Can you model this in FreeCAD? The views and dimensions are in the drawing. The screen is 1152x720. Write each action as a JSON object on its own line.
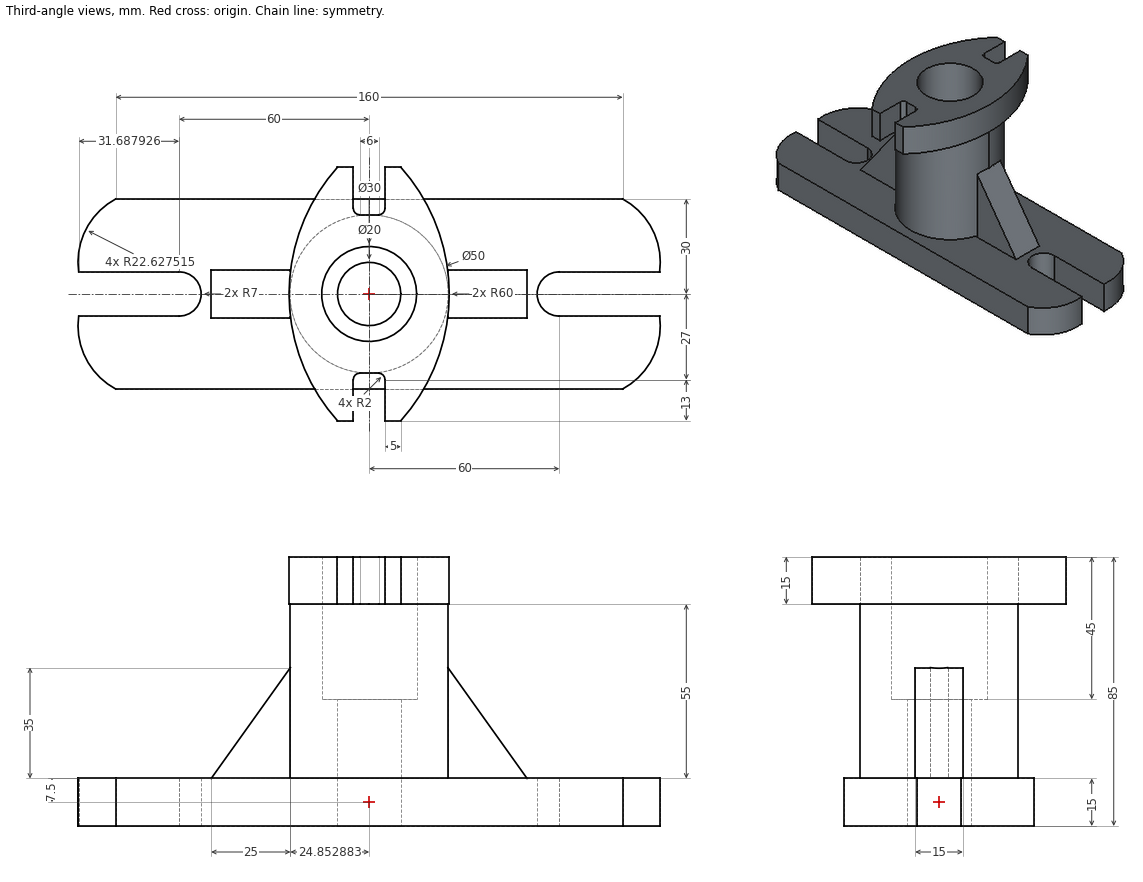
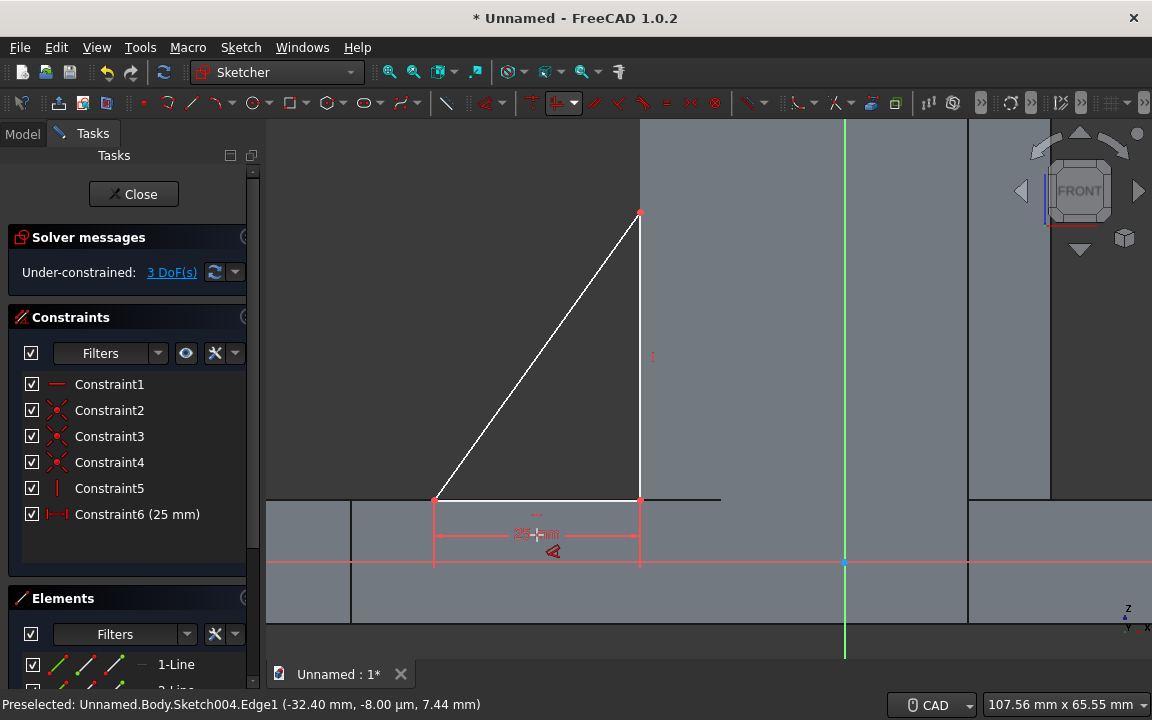
{"action": "left_click", "coordinate": [640, 299]}
{"action": "left_click", "coordinate": [674, 357]}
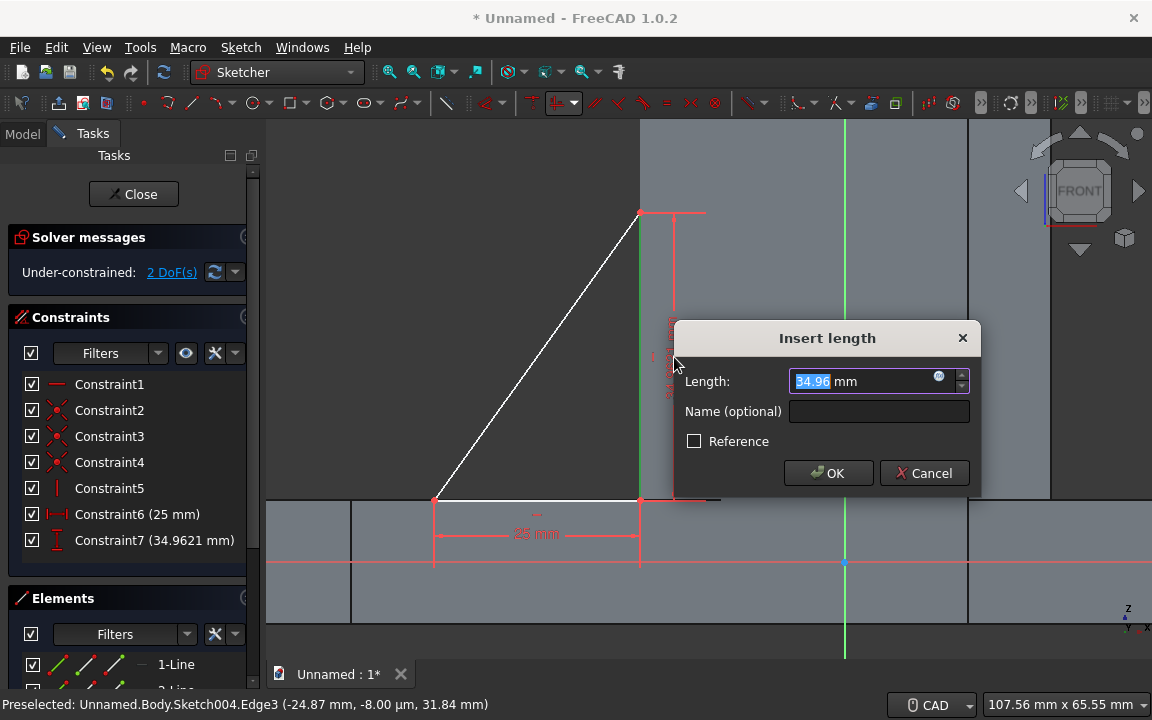
{"action": "type", "text": "35"}
{"action": "key", "text": "Return"}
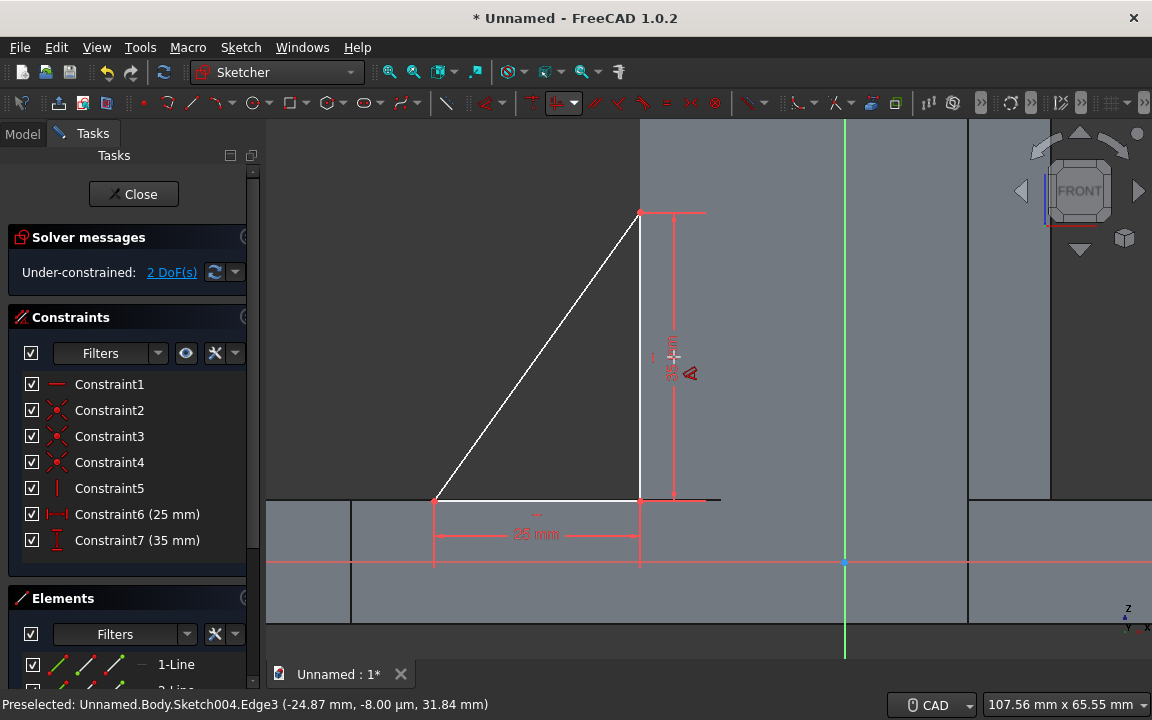
{"action": "left_click", "coordinate": [640, 501]}
{"action": "left_click", "coordinate": [879, 532]}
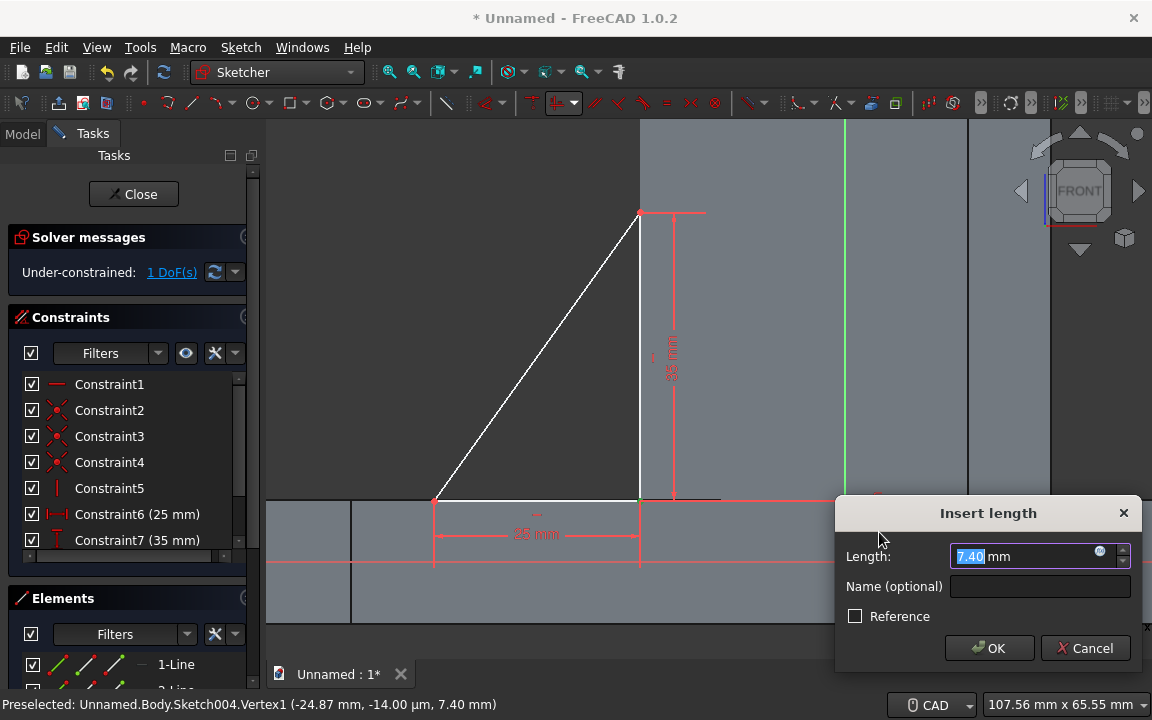
{"action": "type", "text": "7.5"}
{"action": "key", "text": "Return"}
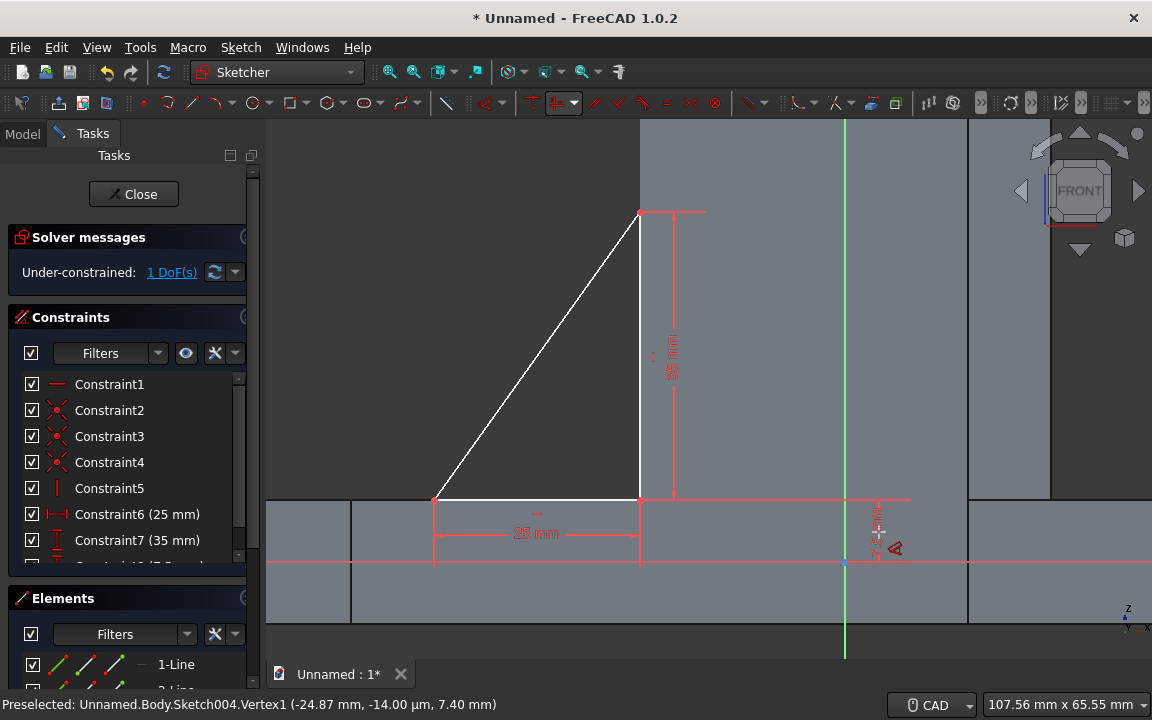
{"action": "left_click", "coordinate": [640, 500]}
{"action": "left_click", "coordinate": [742, 596]}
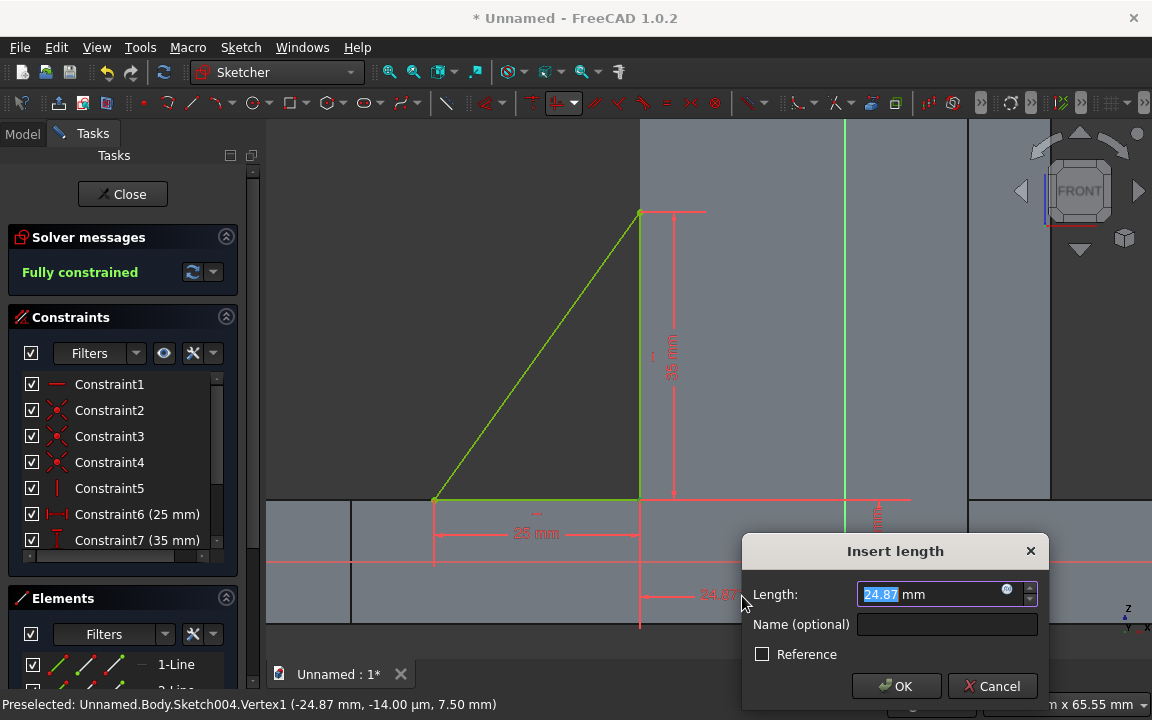
{"action": "type", "text": "24.852883"}
{"action": "key", "text": "Return"}
{"action": "key", "text": "Escape"}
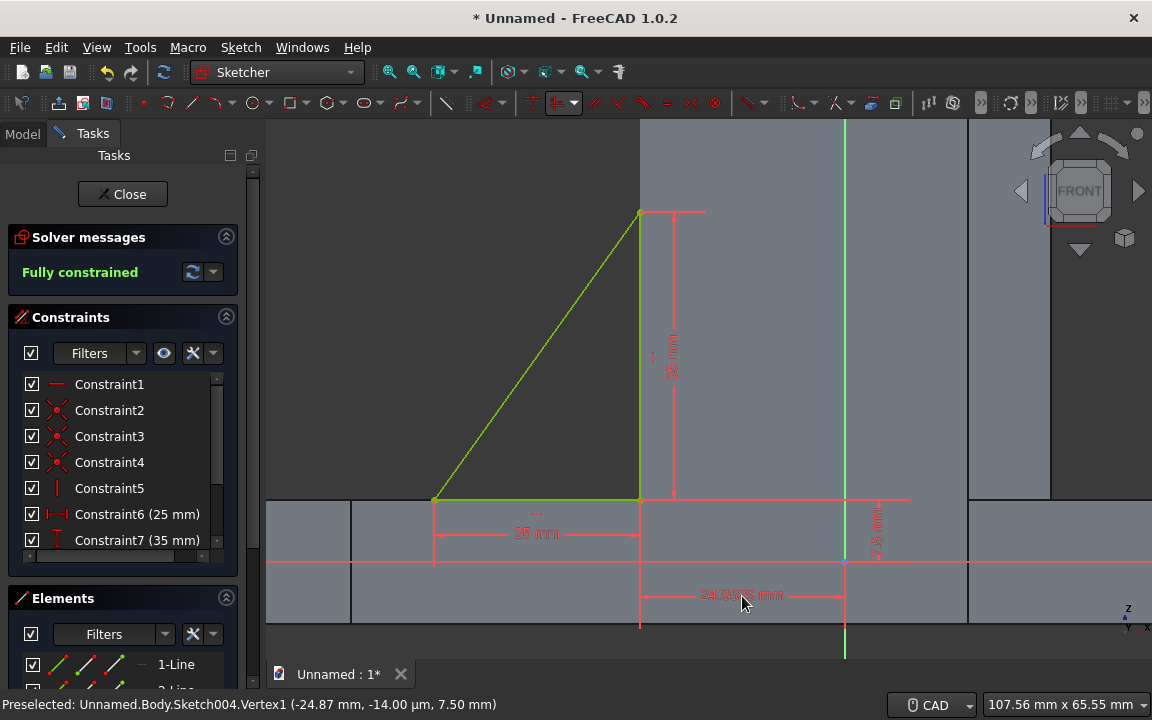
{"action": "left_click", "coordinate": [123, 194]}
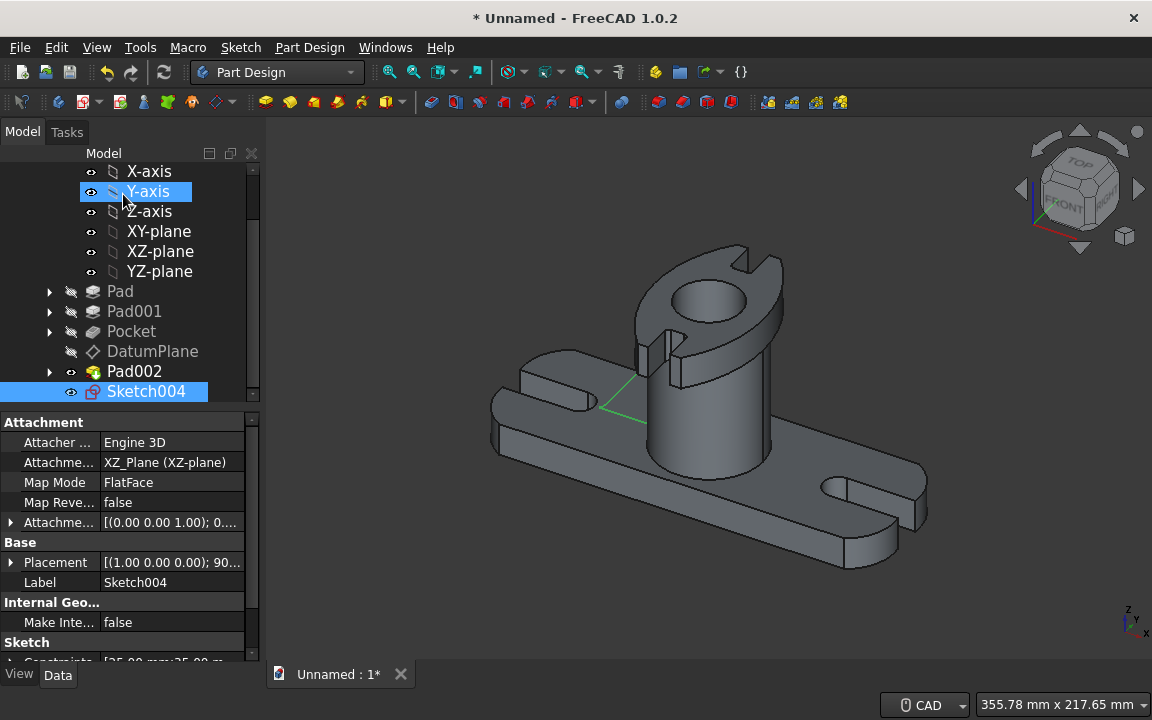
{"action": "left_click", "coordinate": [266, 102]}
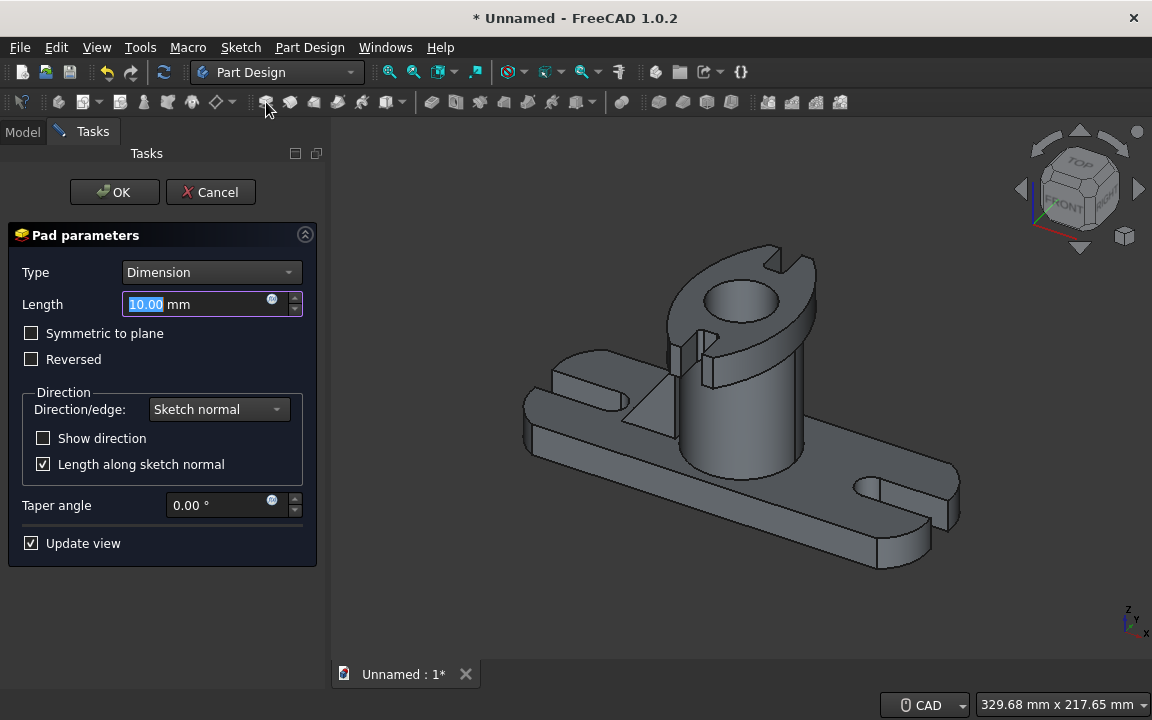
{"action": "type", "text": "15"}
{"action": "key", "text": "Tab"}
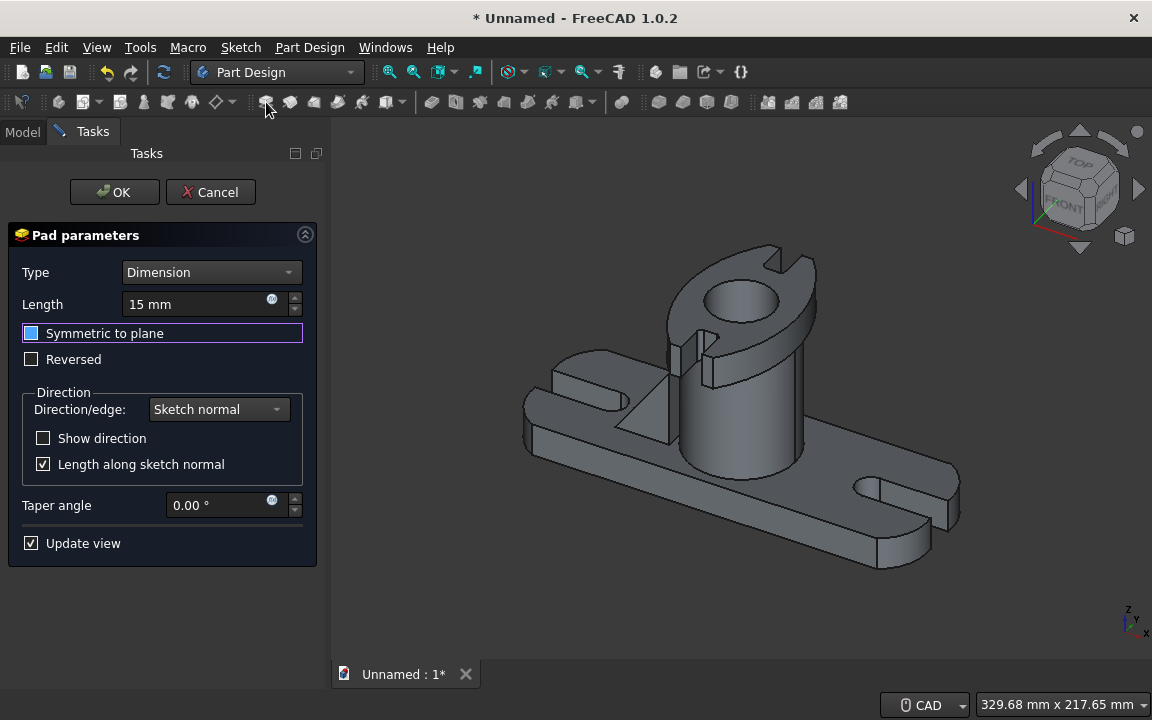
{"action": "left_click", "coordinate": [30, 333]}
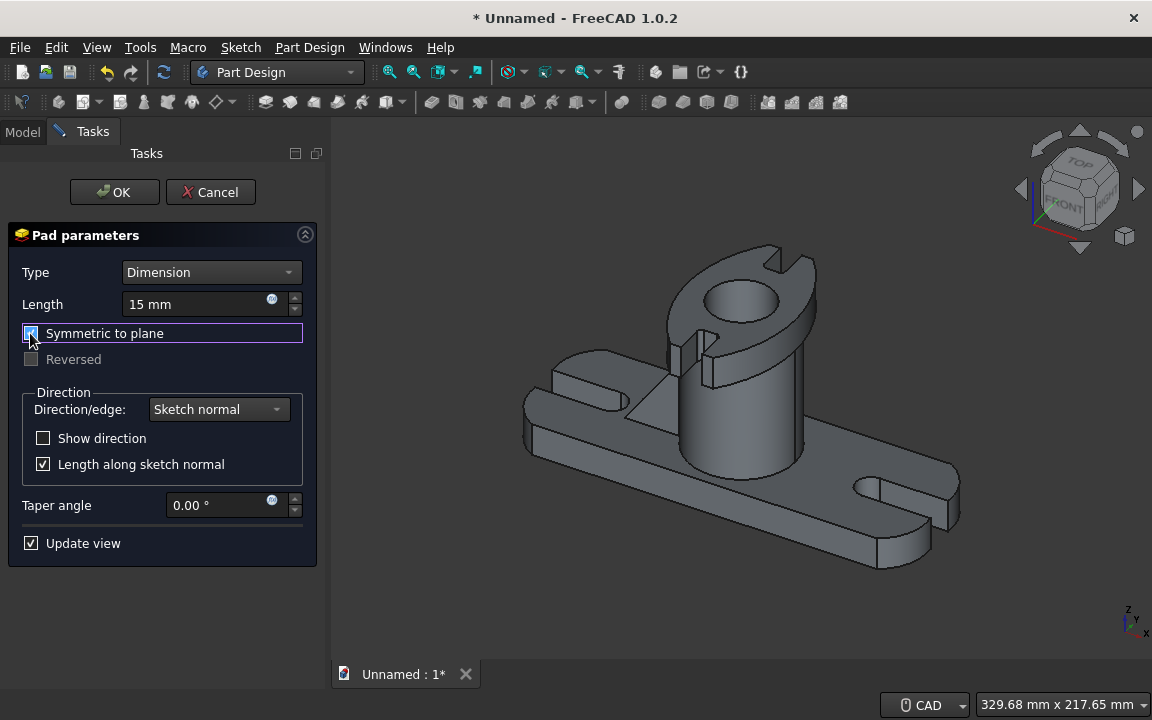
{"action": "left_click", "coordinate": [115, 192]}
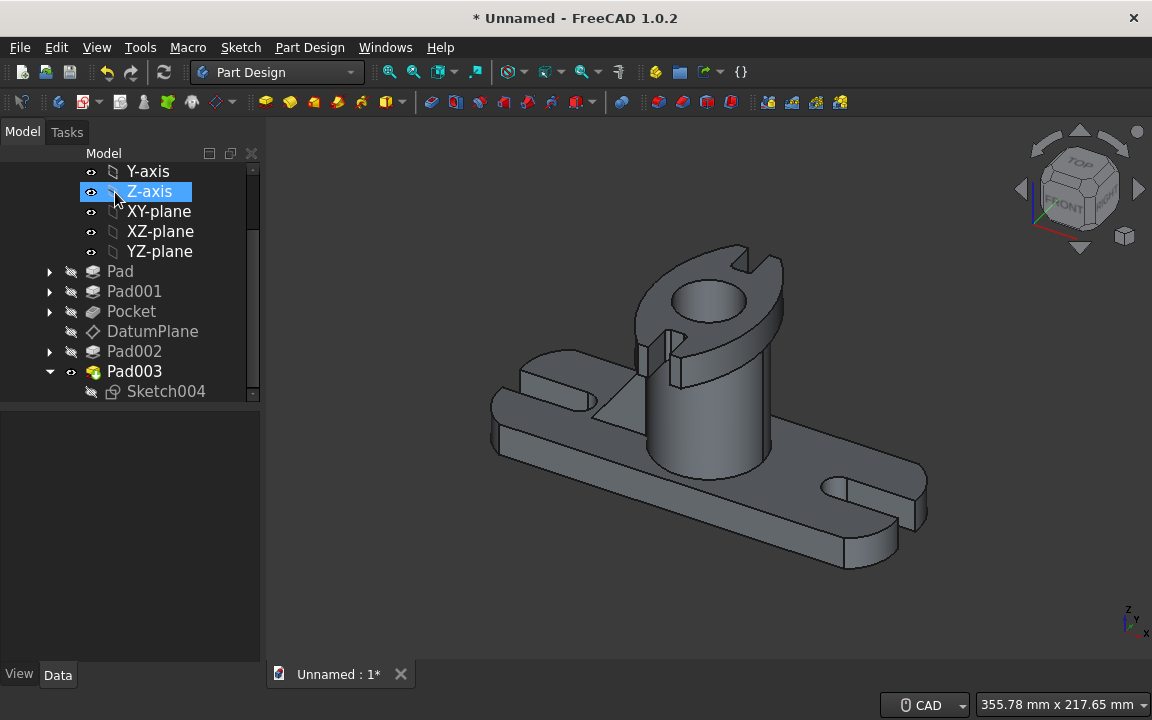
{"action": "left_click", "coordinate": [116, 372]}